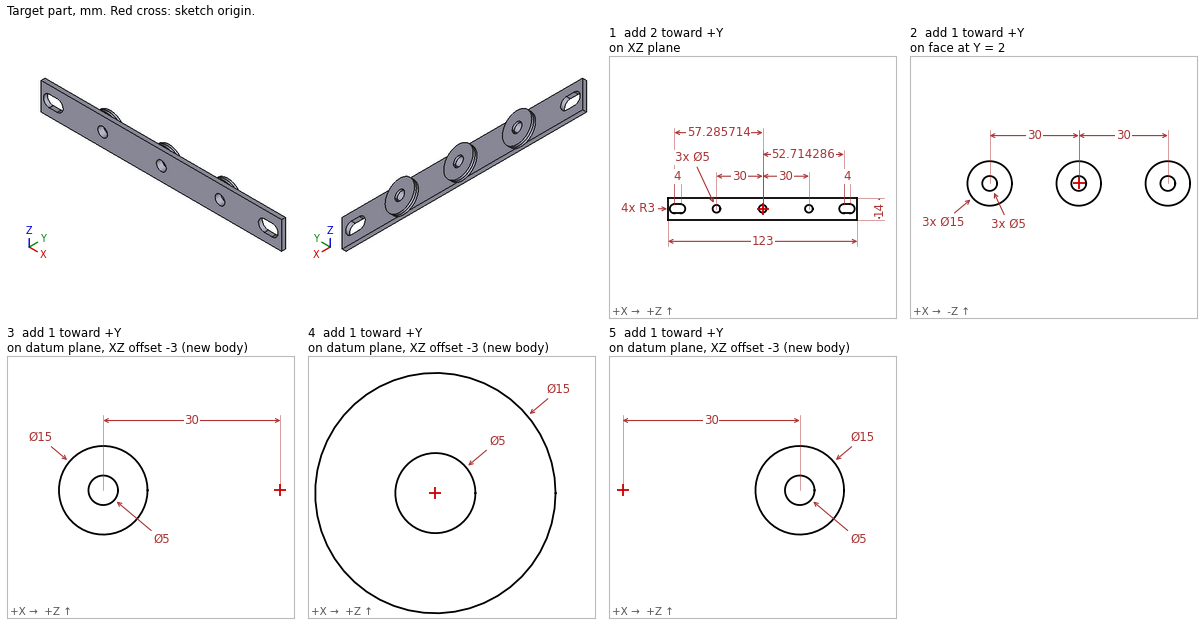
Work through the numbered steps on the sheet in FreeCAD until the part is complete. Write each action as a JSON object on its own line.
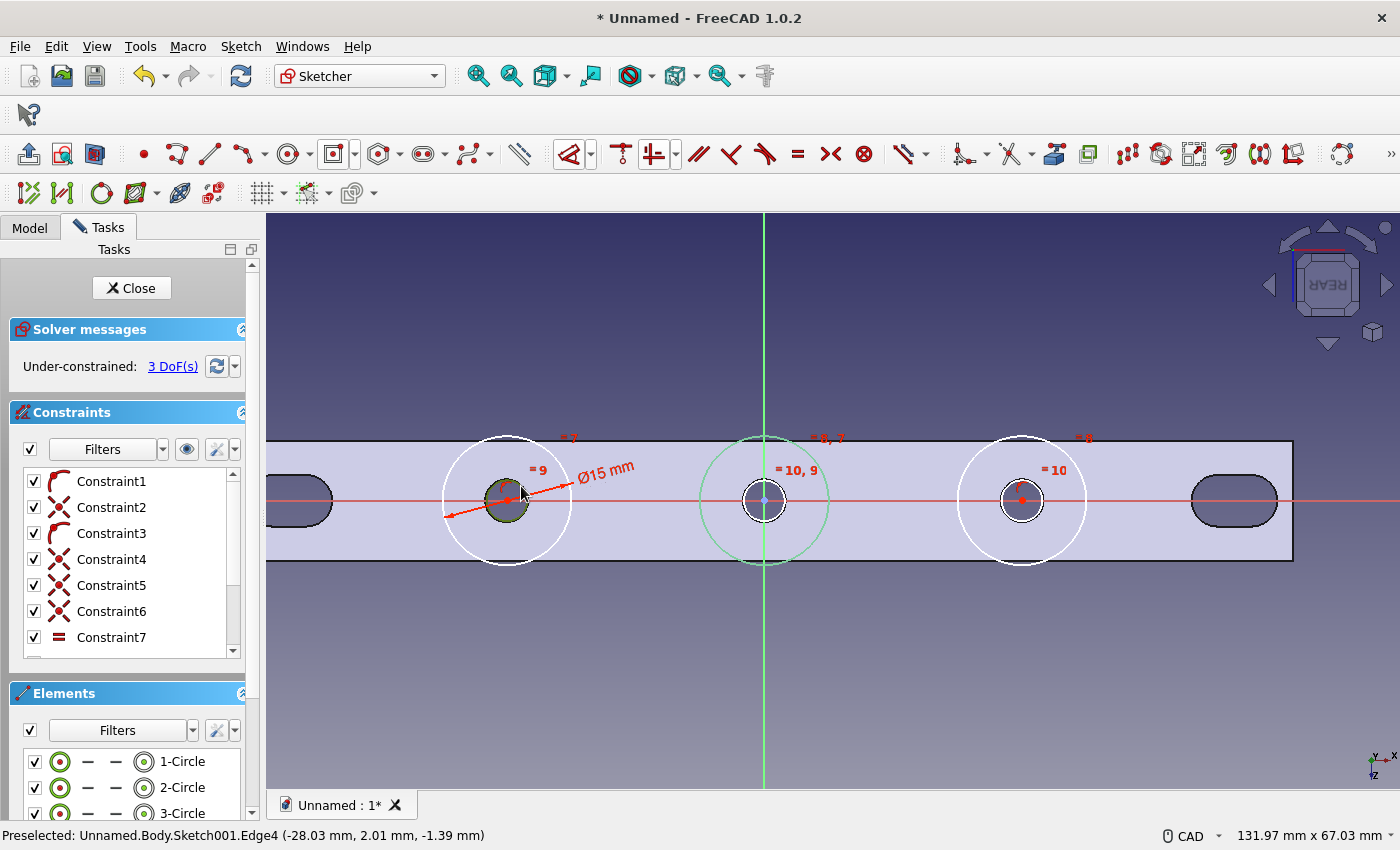
{"action": "key", "text": "k o"}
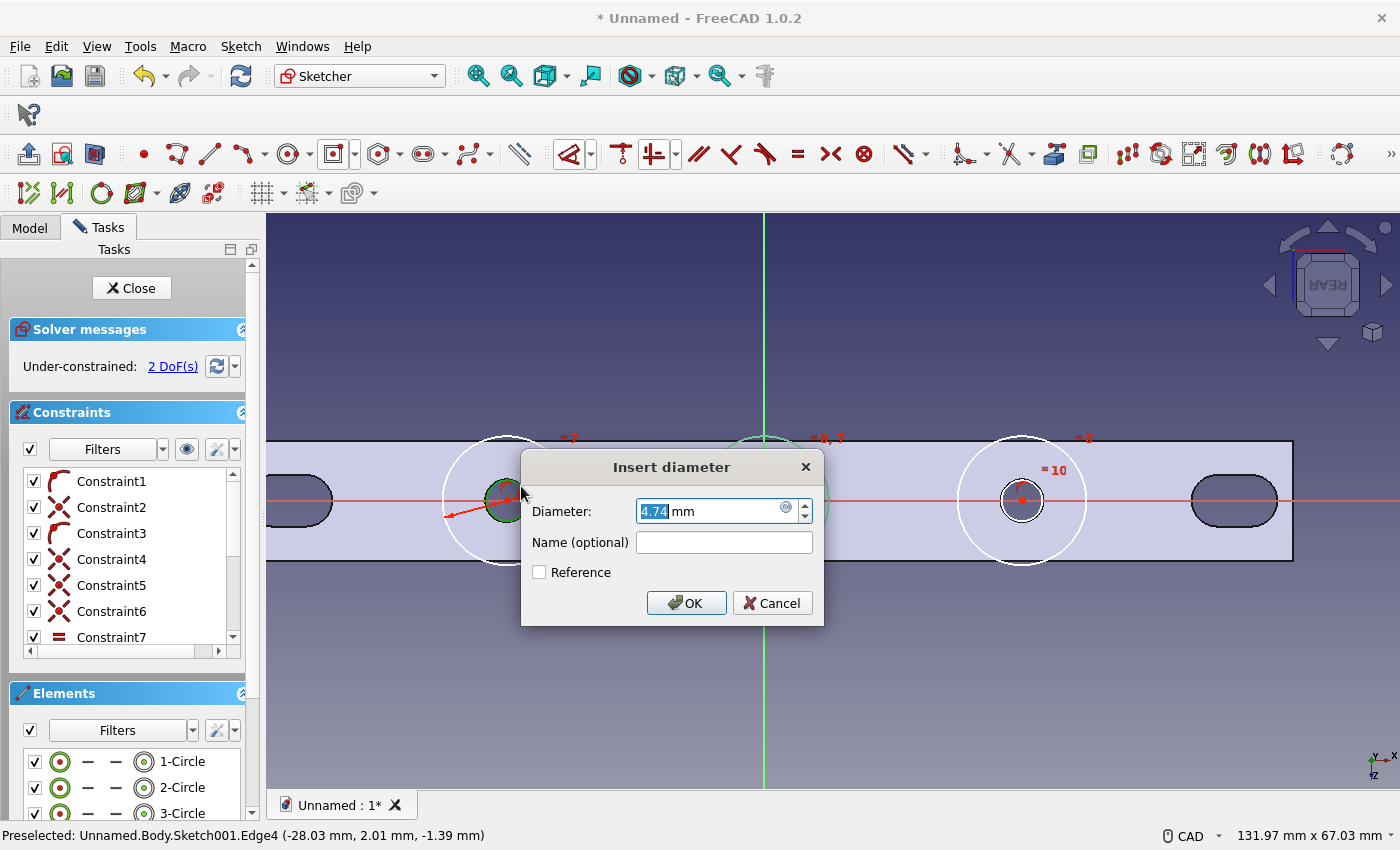
{"action": "type", "text": "5"}
{"action": "key", "text": "Return"}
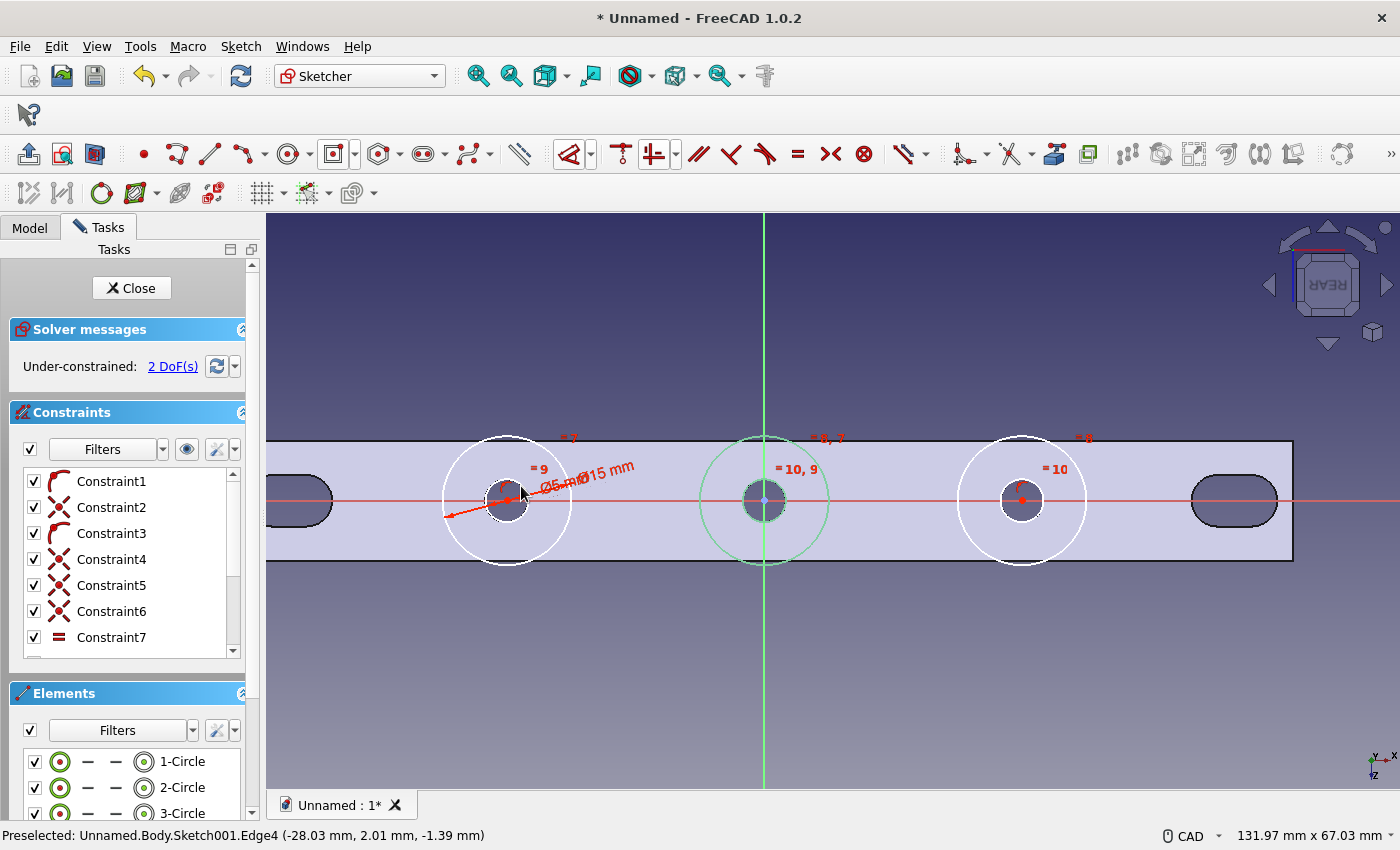
{"action": "left_click", "coordinate": [507, 501]}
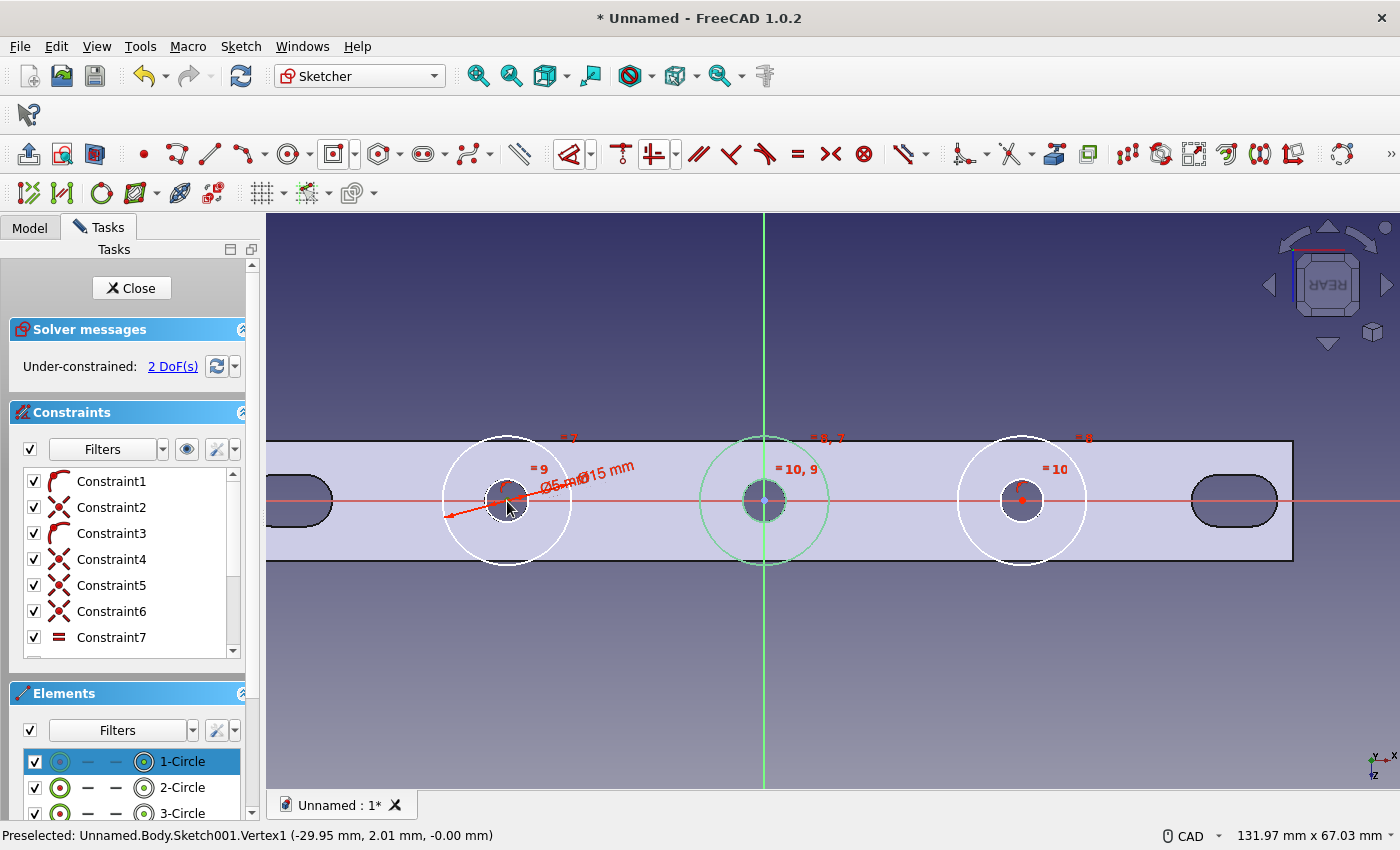
{"action": "left_click", "coordinate": [590, 154]}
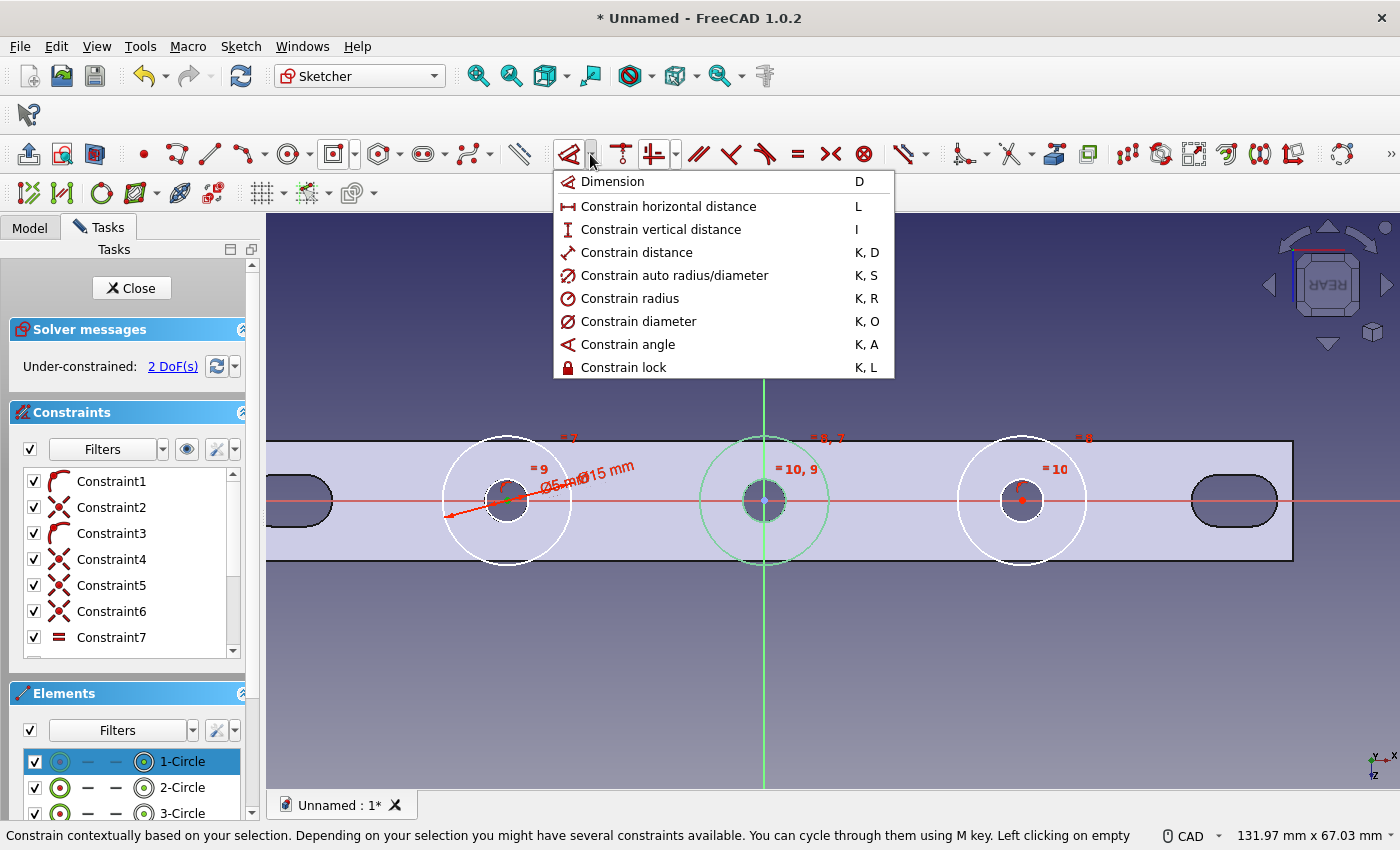
{"action": "left_click", "coordinate": [724, 206]}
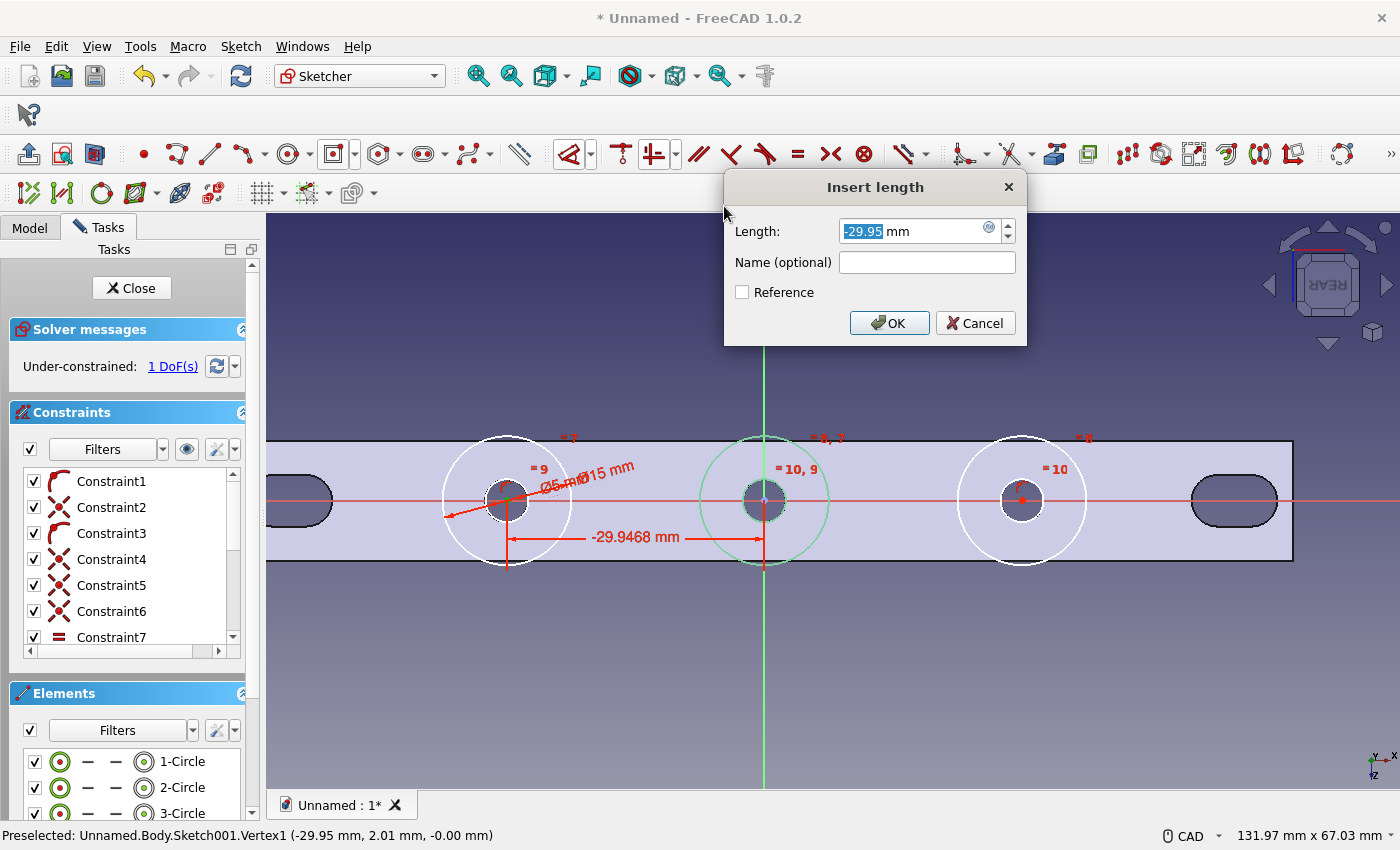
{"action": "type", "text": "-30"}
{"action": "key", "text": "Return"}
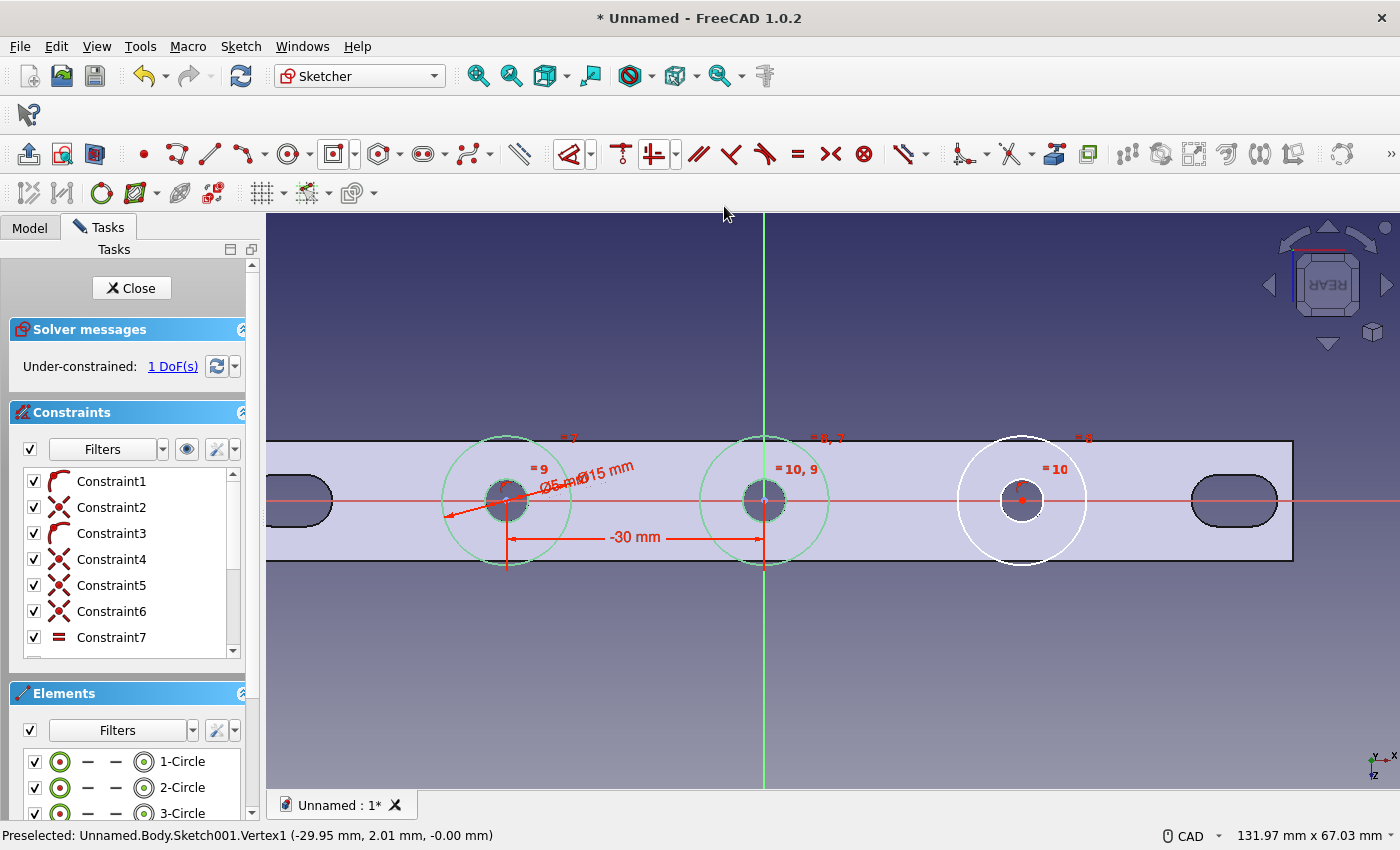
{"action": "left_click", "coordinate": [1022, 501]}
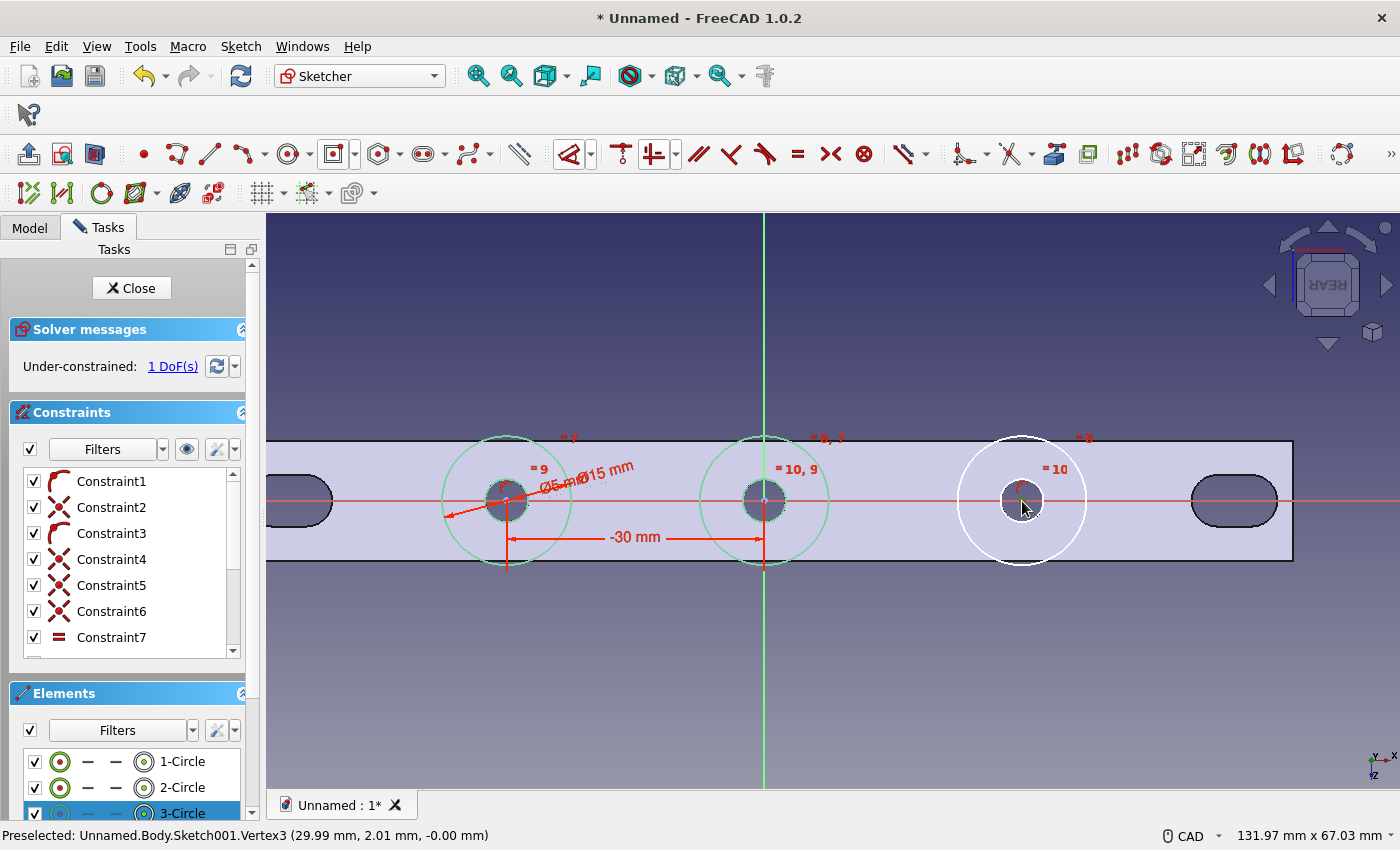
{"action": "key", "text": "l"}